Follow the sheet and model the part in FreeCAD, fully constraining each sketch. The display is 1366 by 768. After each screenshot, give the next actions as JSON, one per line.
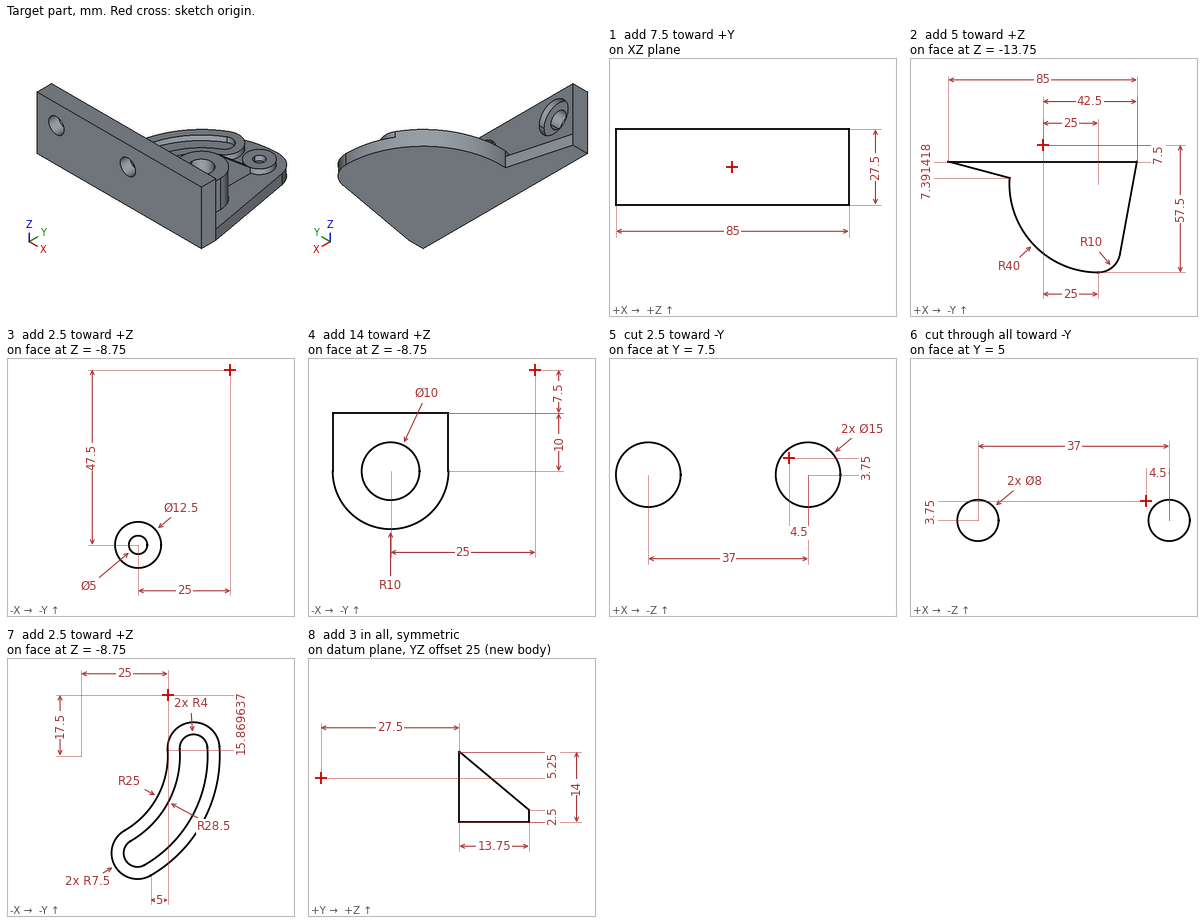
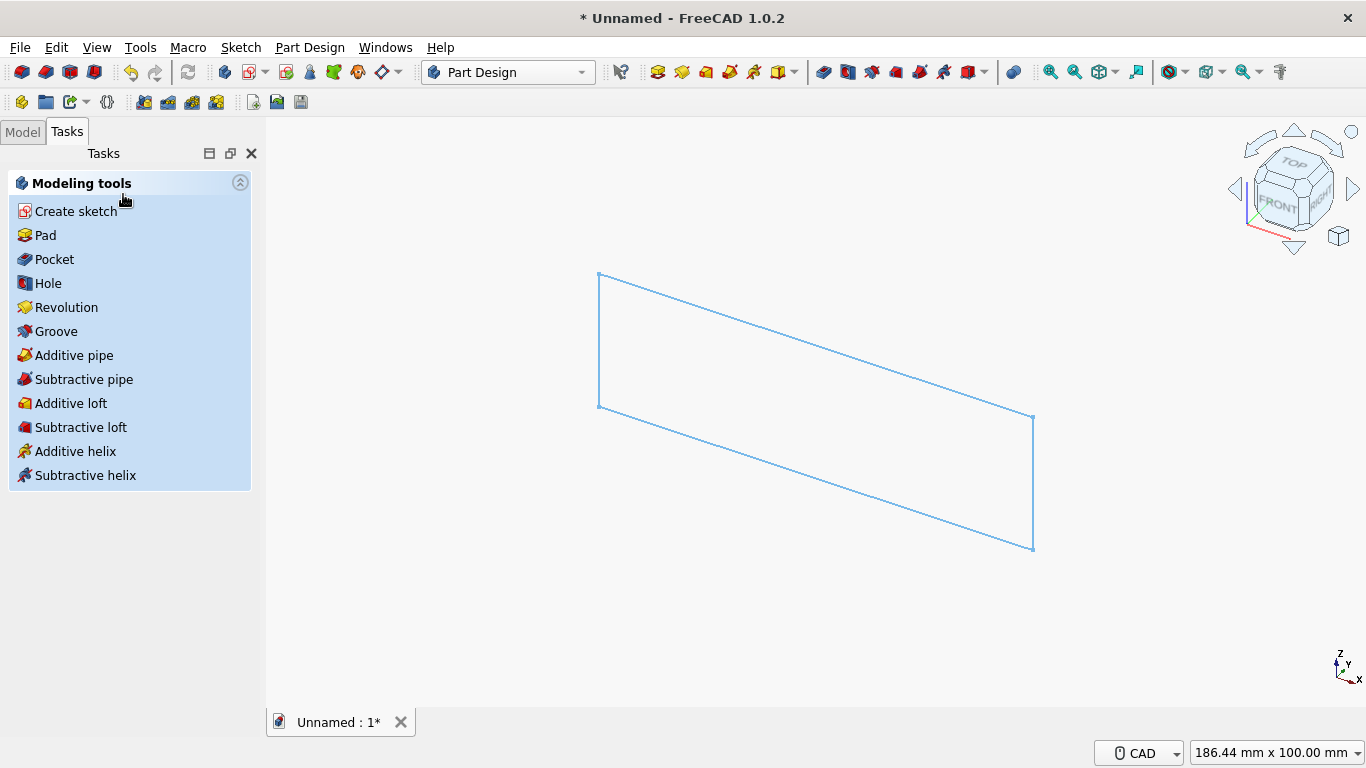
{"action": "left_click", "coordinate": [658, 72]}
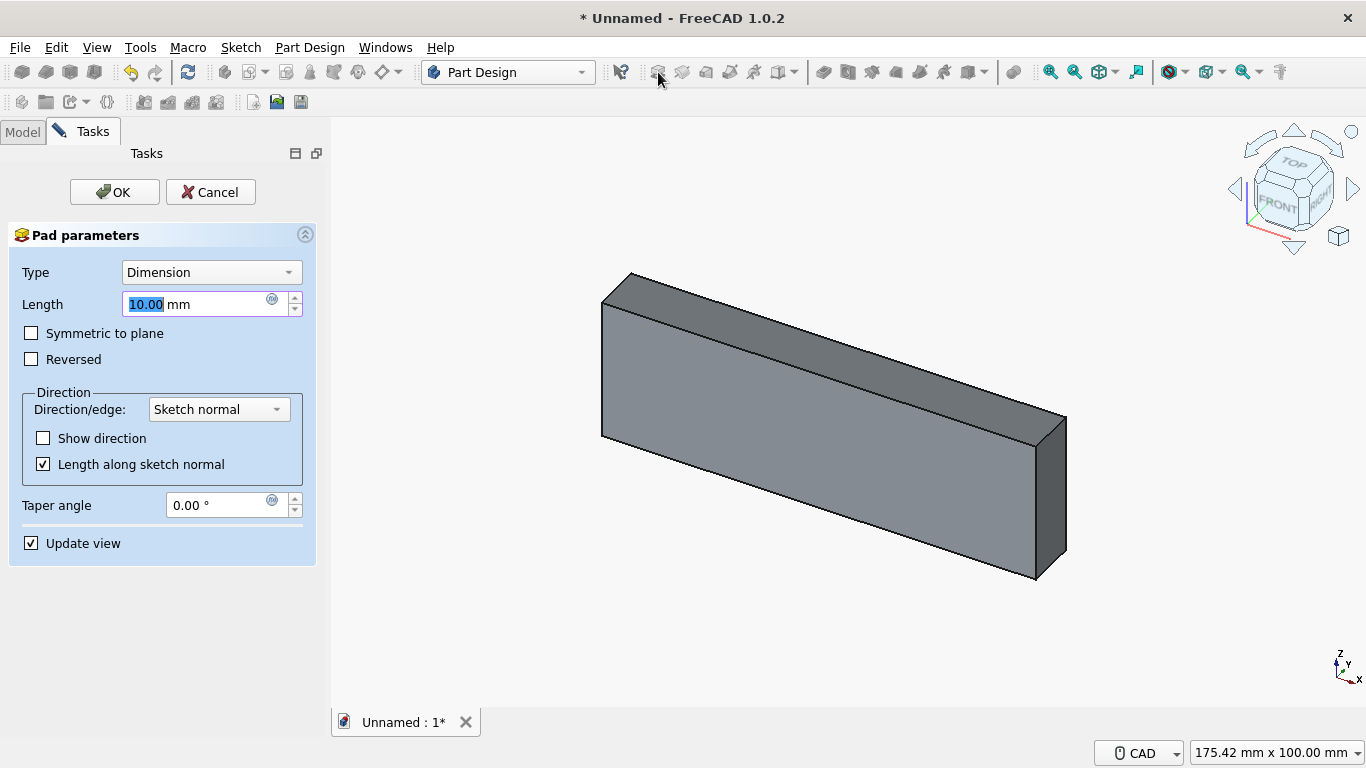
{"action": "type", "text": "7.5"}
{"action": "key", "text": "Tab"}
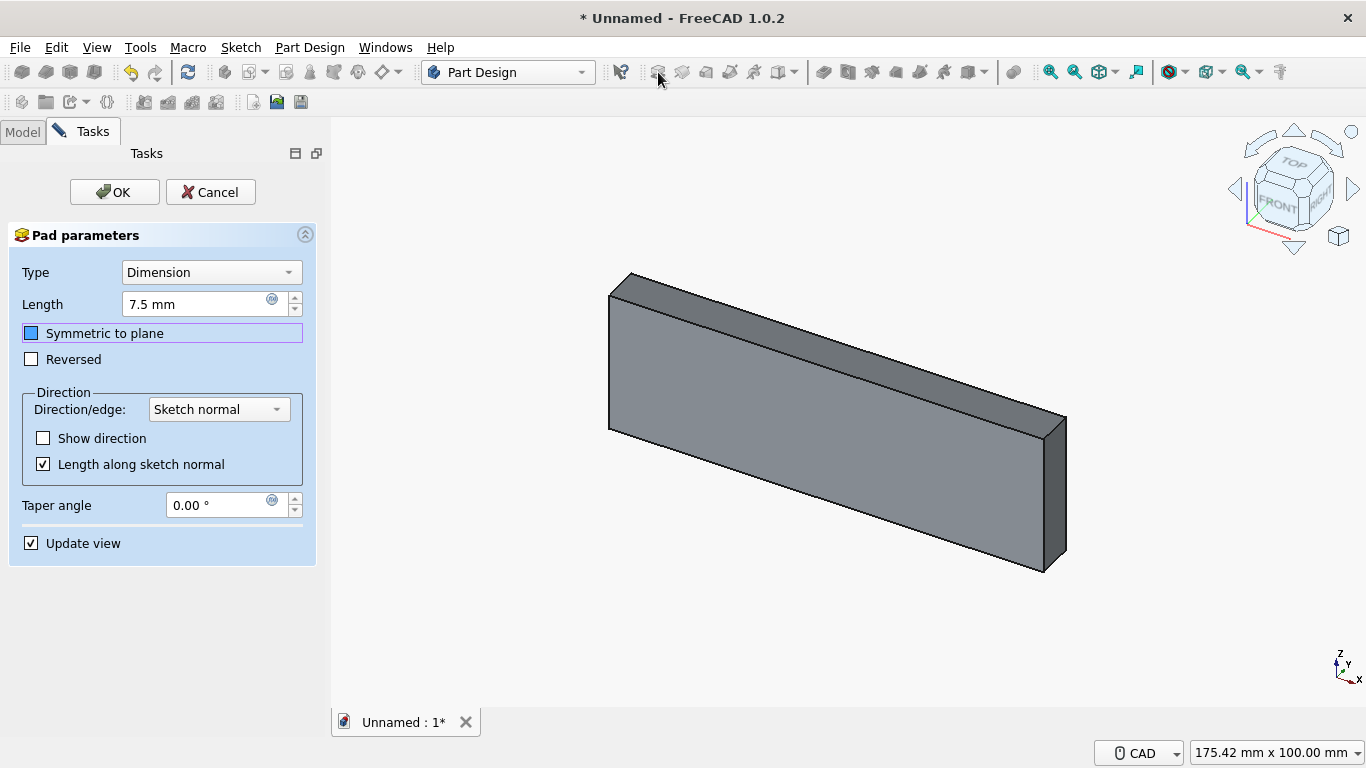
{"action": "left_click", "coordinate": [30, 359]}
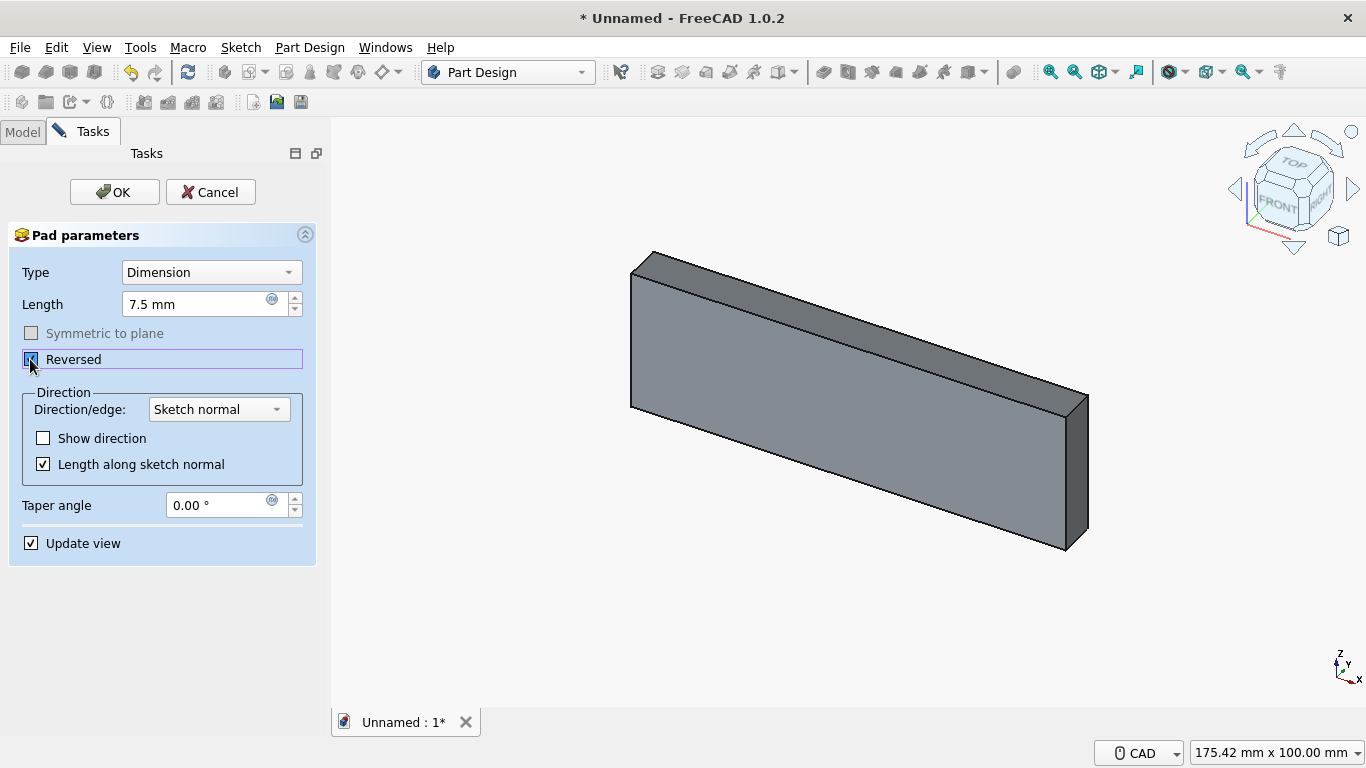
{"action": "left_click", "coordinate": [115, 192]}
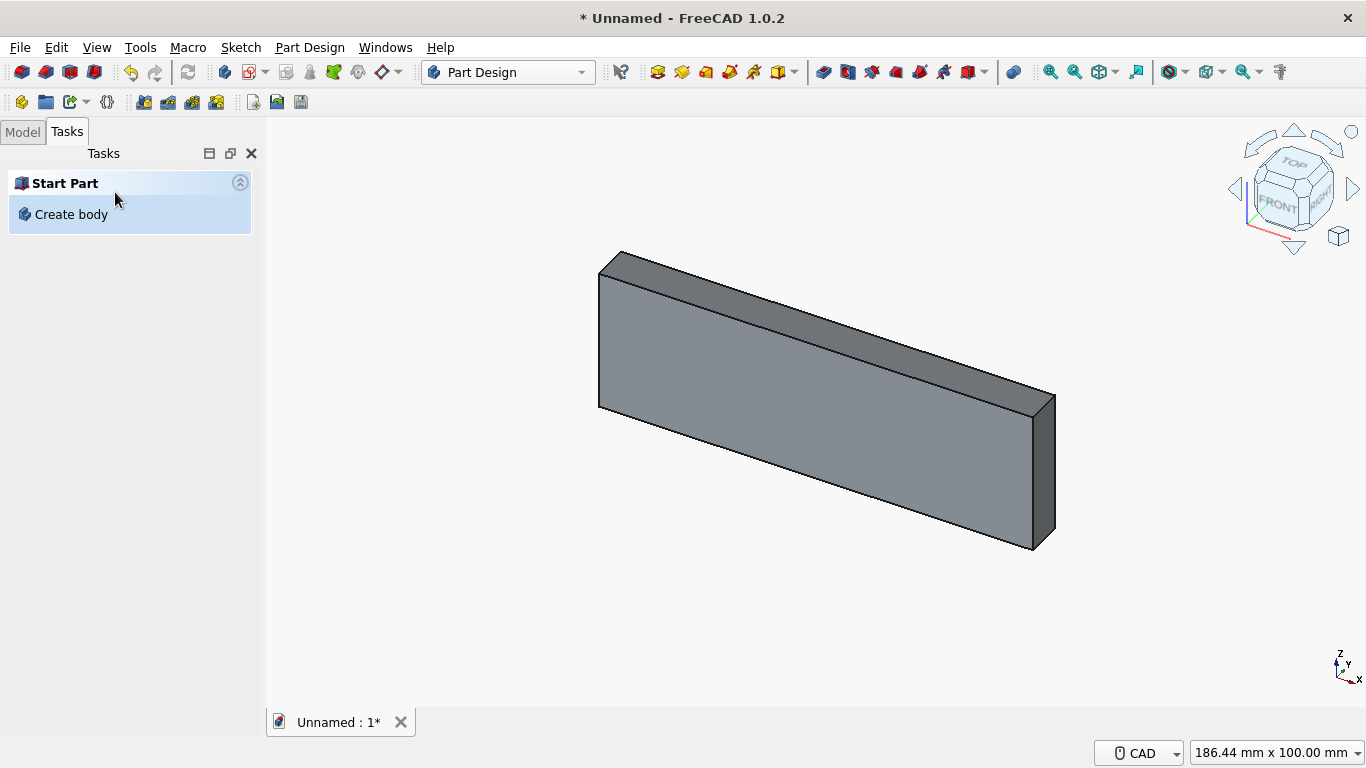
{"action": "key", "text": "5"}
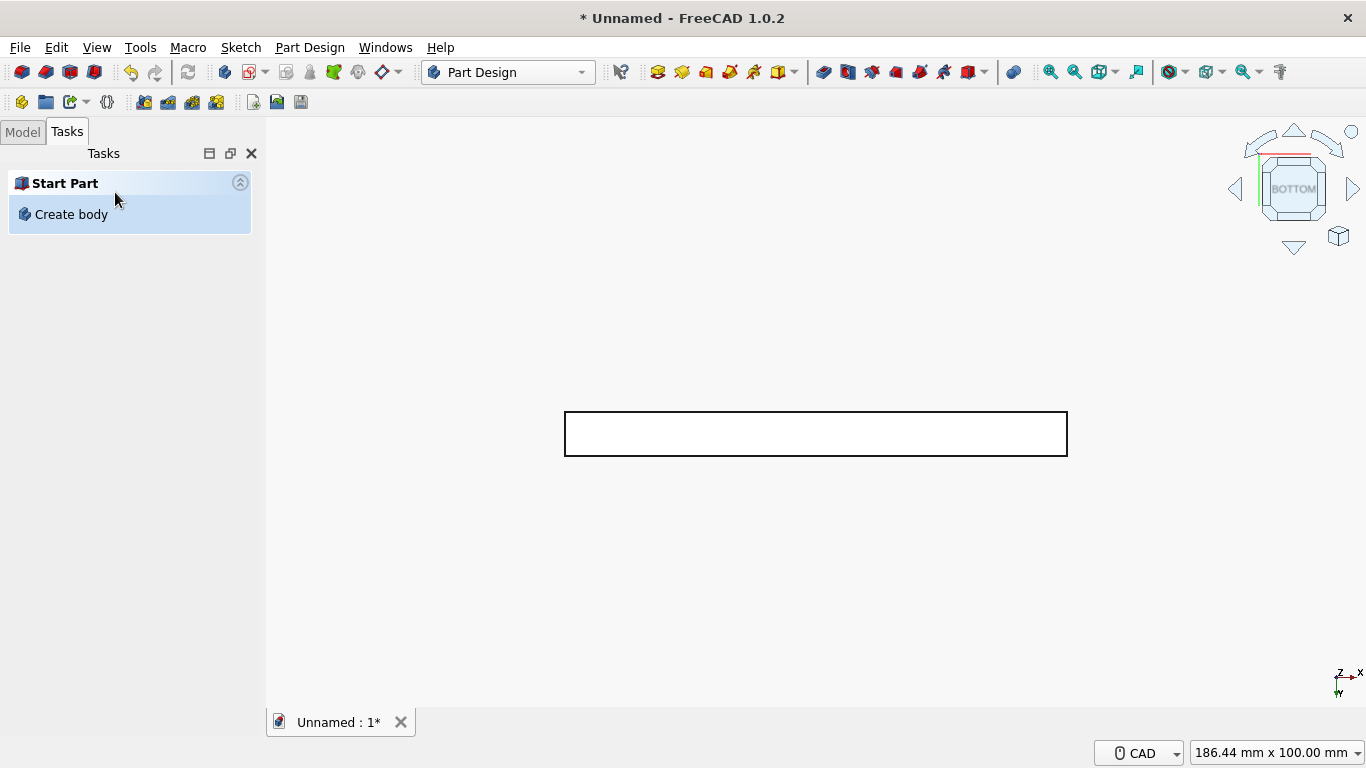
{"action": "left_click", "coordinate": [1031, 433]}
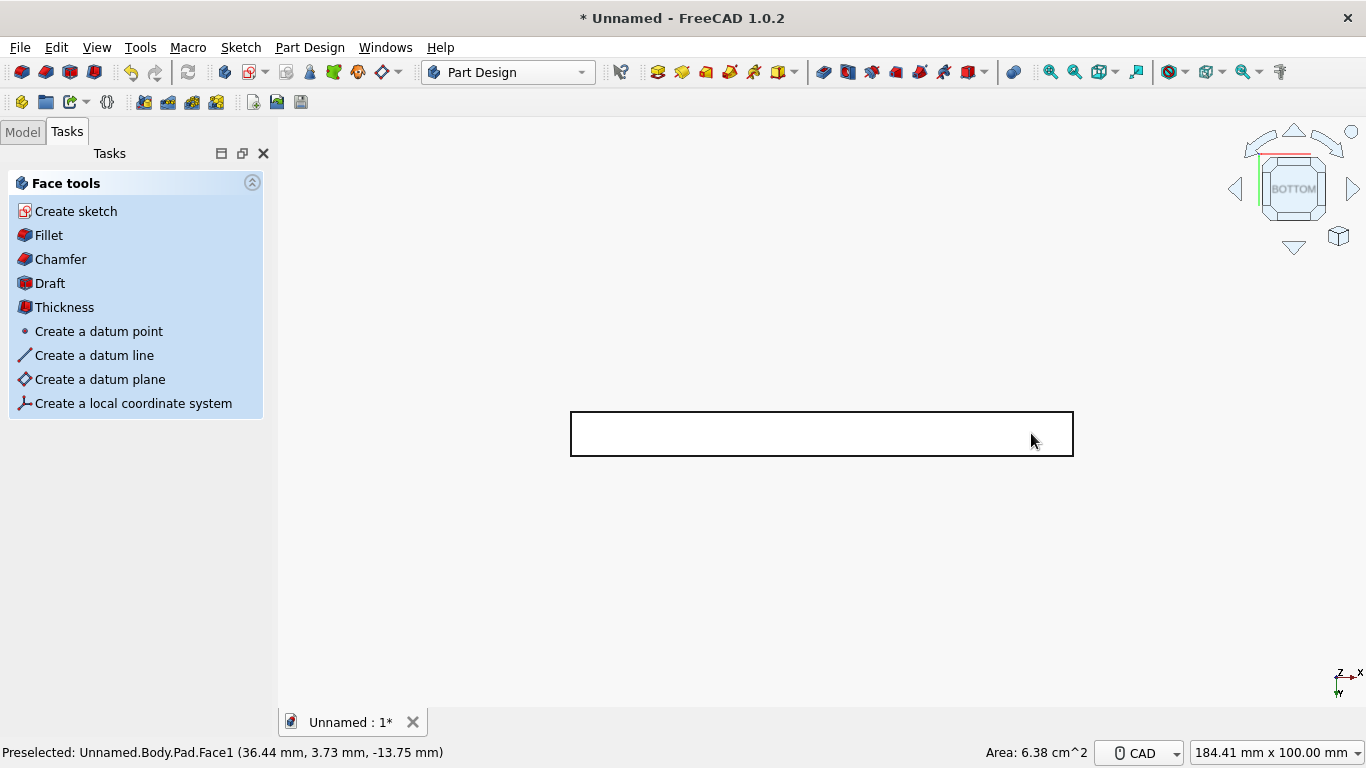
{"action": "left_click", "coordinate": [250, 72]}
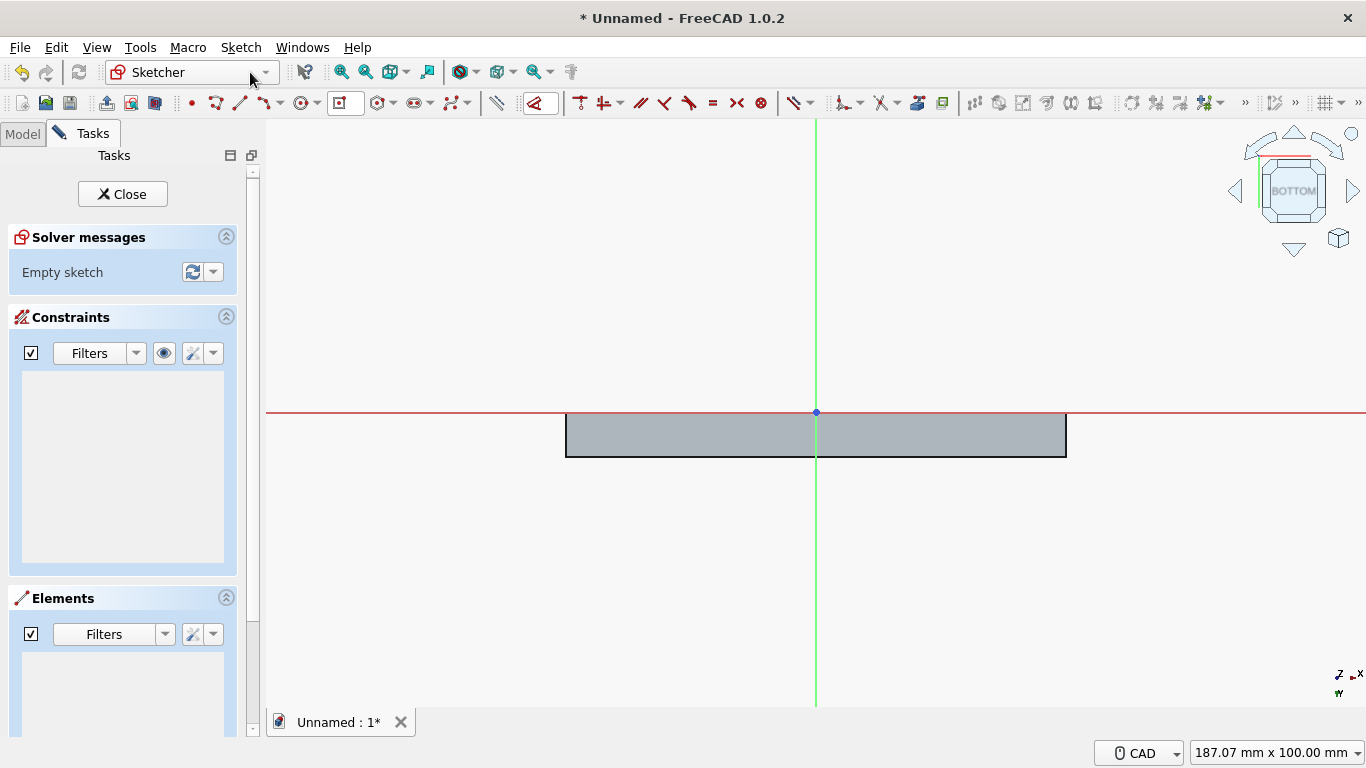
{"action": "scroll", "coordinate": [438, 147], "scroll_direction": "down", "scroll_amount": 1}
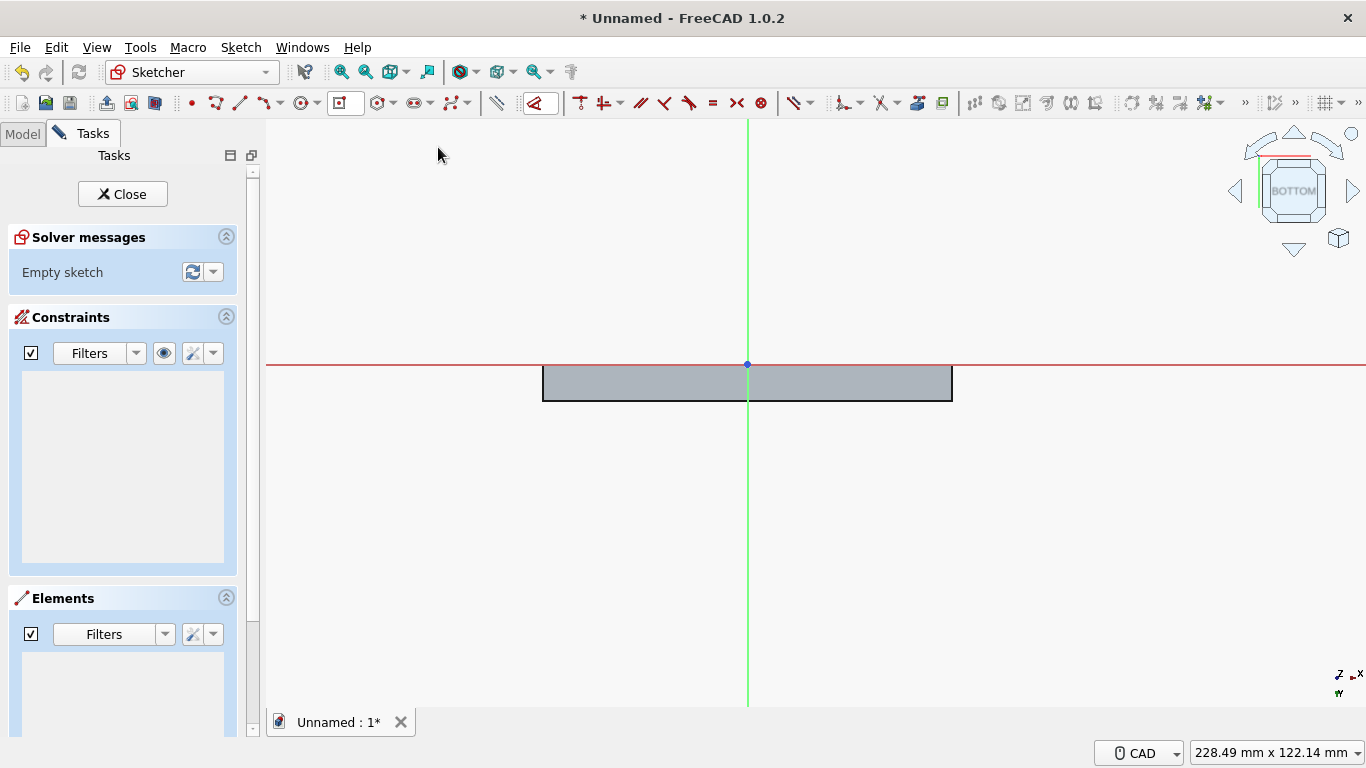
{"action": "scroll", "coordinate": [748, 679], "scroll_direction": "up", "scroll_amount": 2}